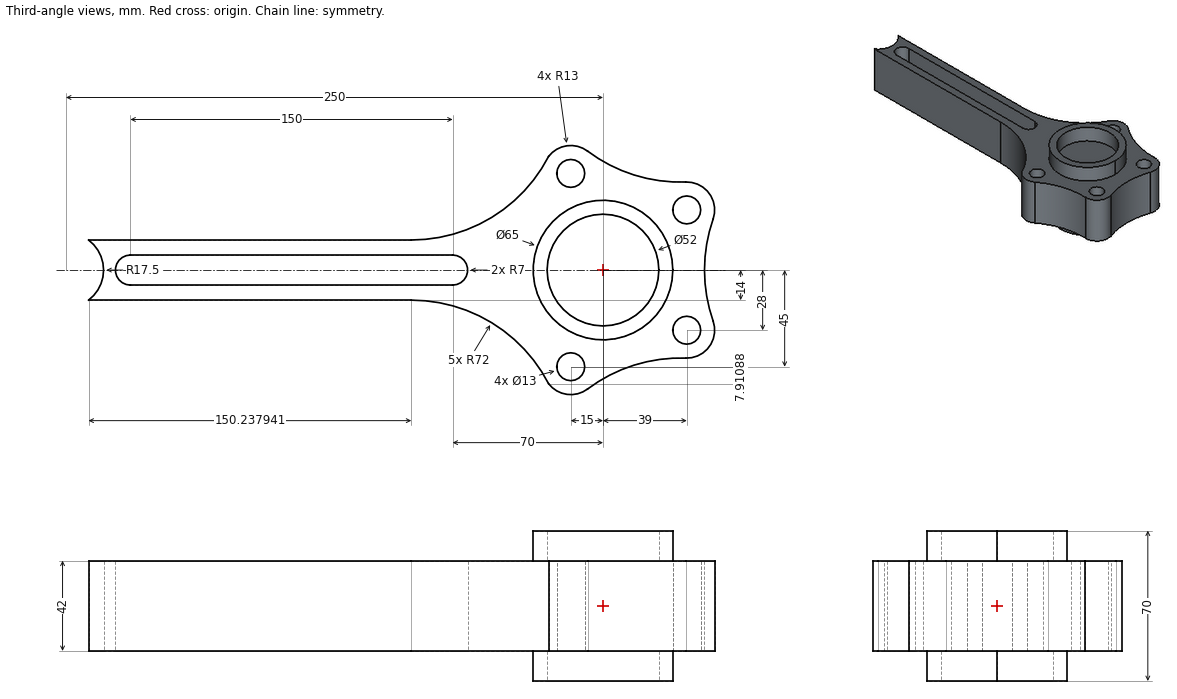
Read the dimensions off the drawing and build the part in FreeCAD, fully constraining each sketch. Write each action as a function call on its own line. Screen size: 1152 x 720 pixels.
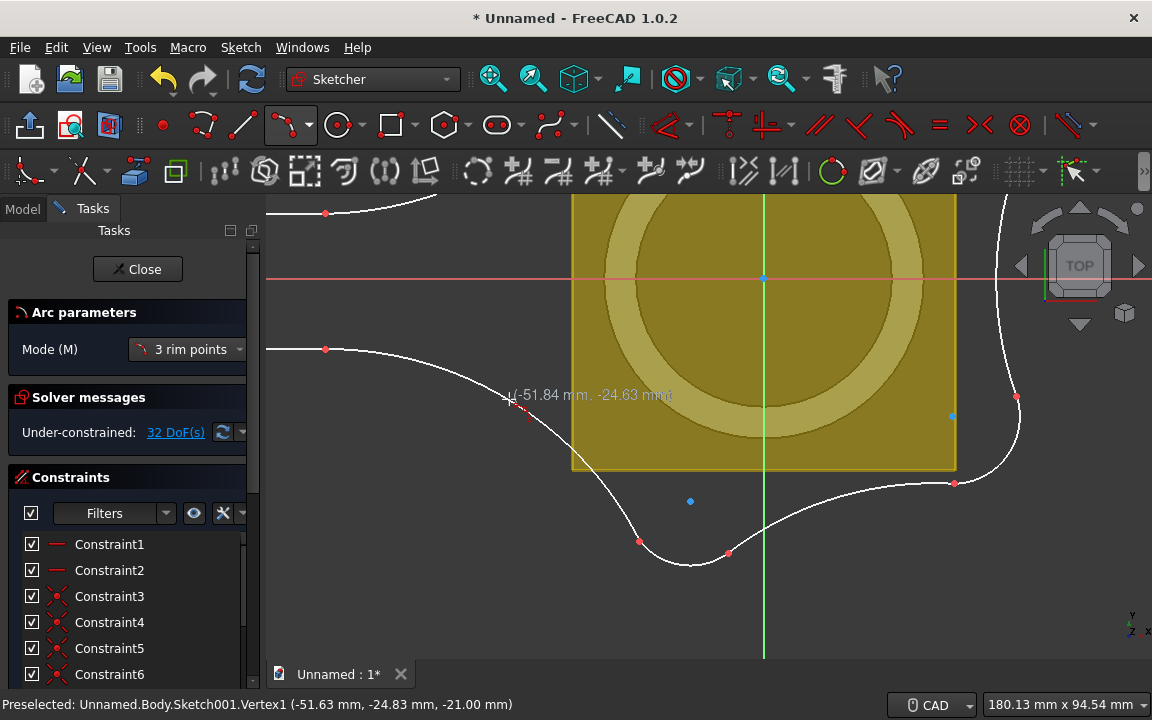
click(498, 126)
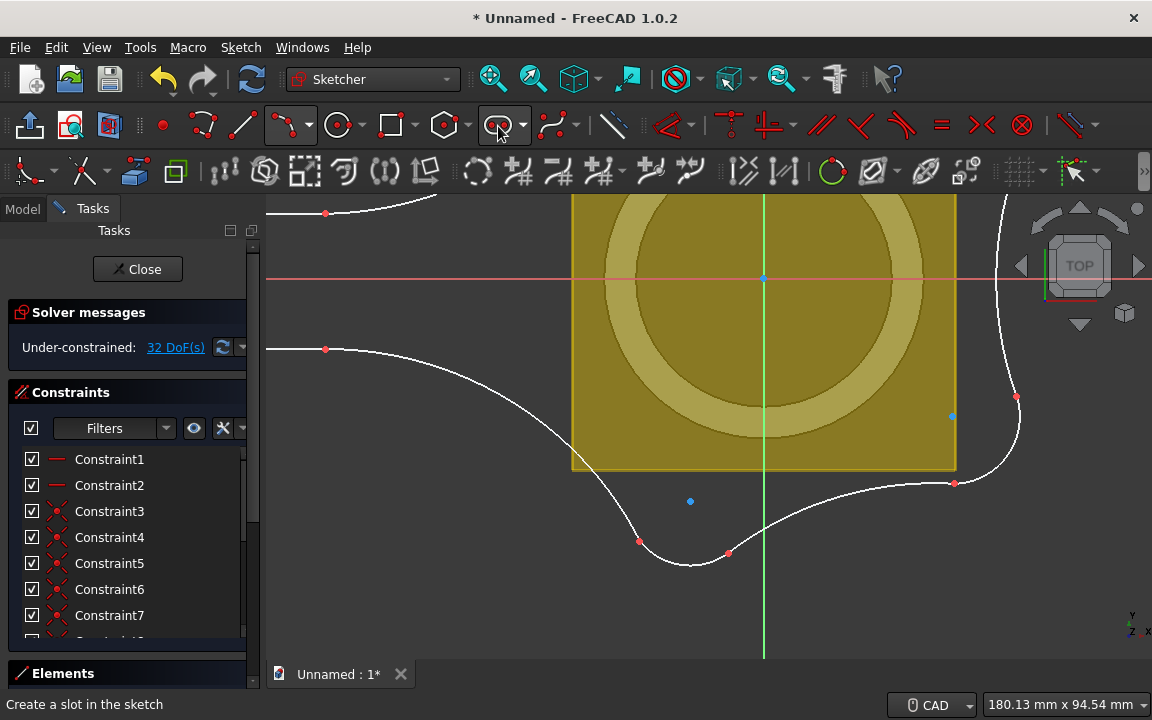
scroll(838, 512, down, 5)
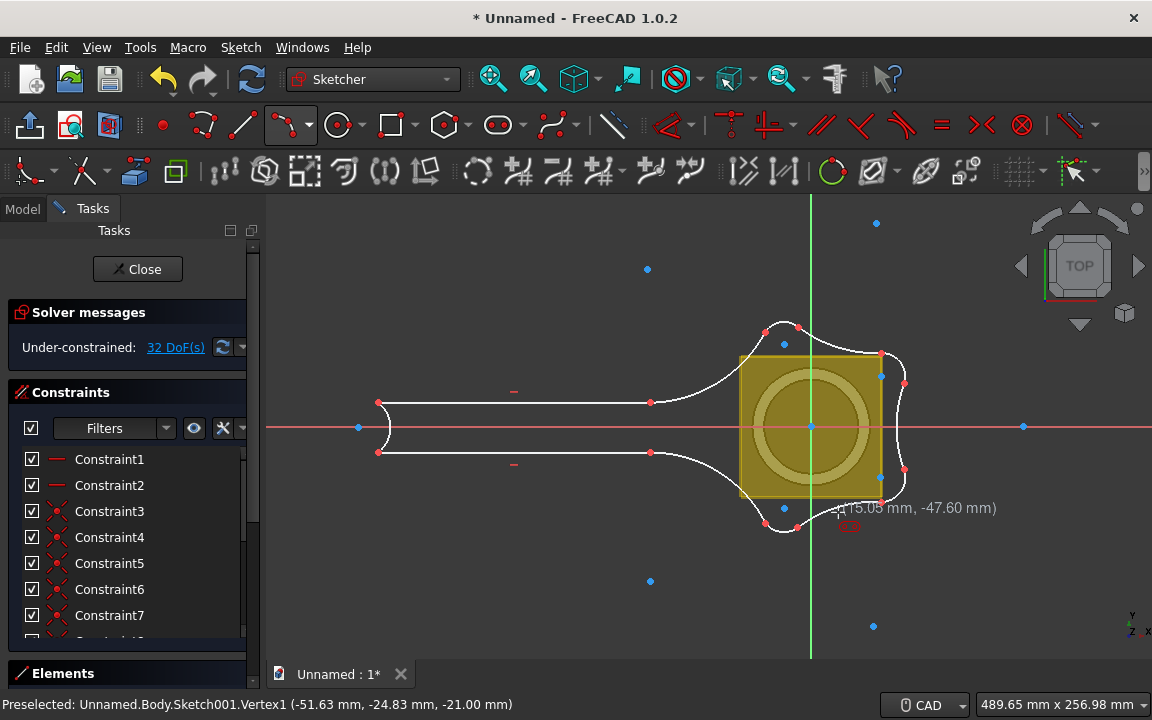
scroll(413, 427, up, 3)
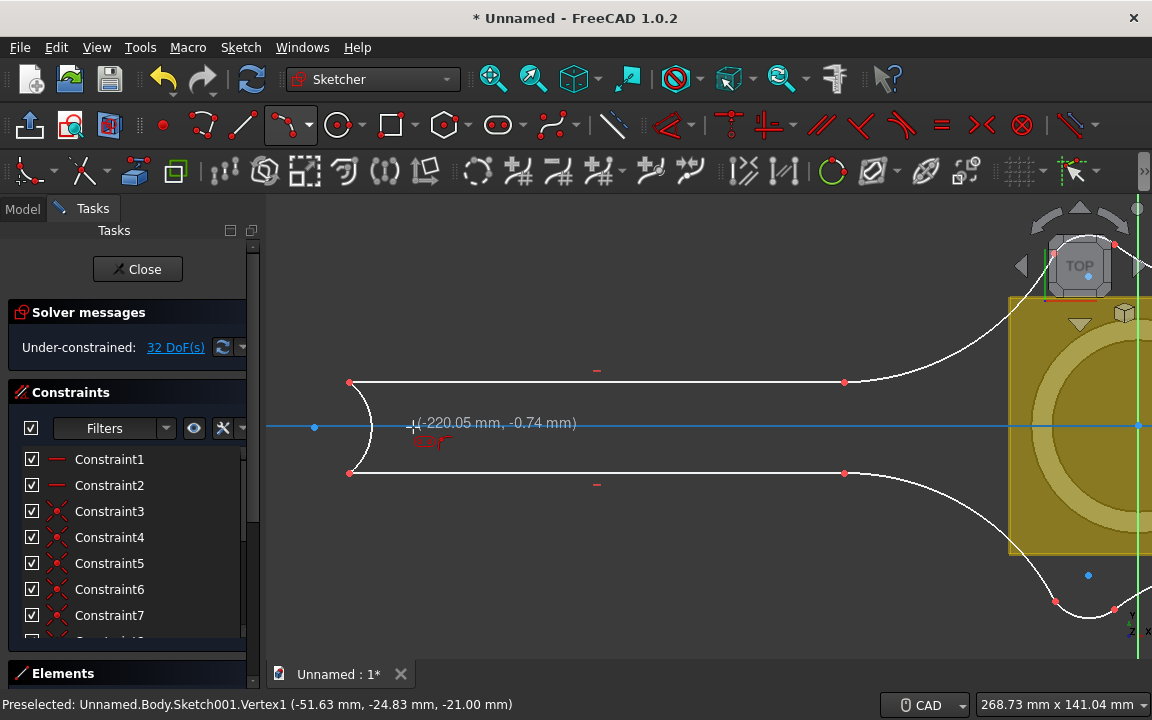
click(413, 426)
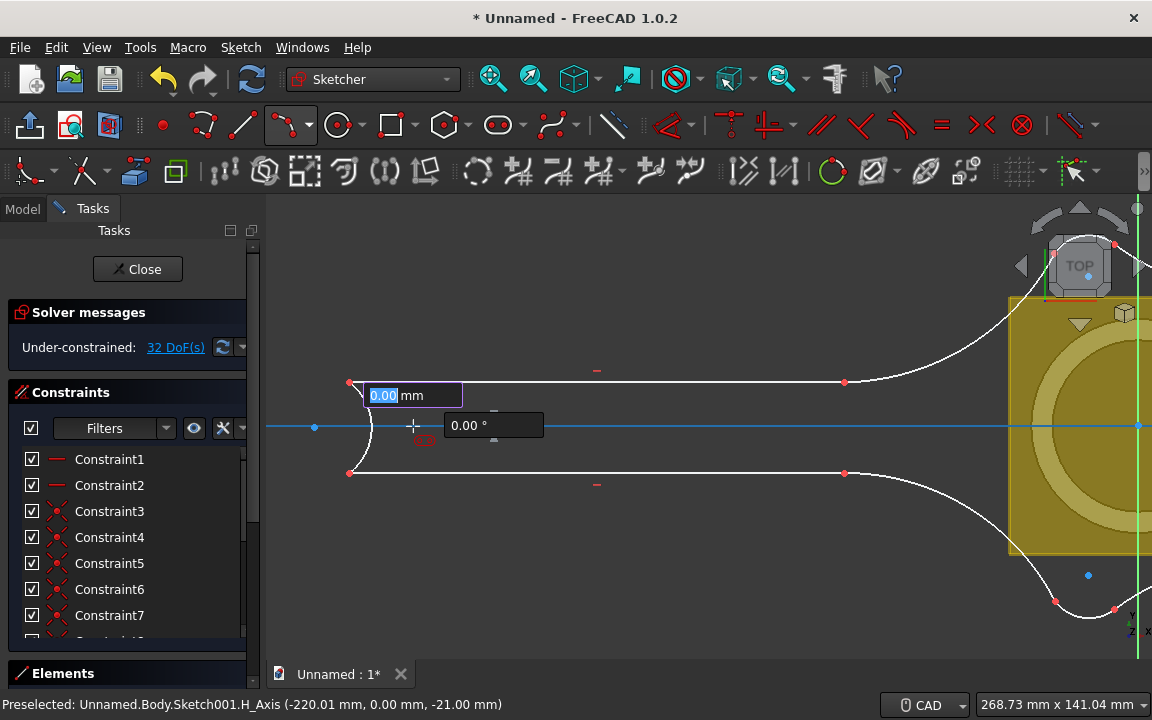
click(908, 417)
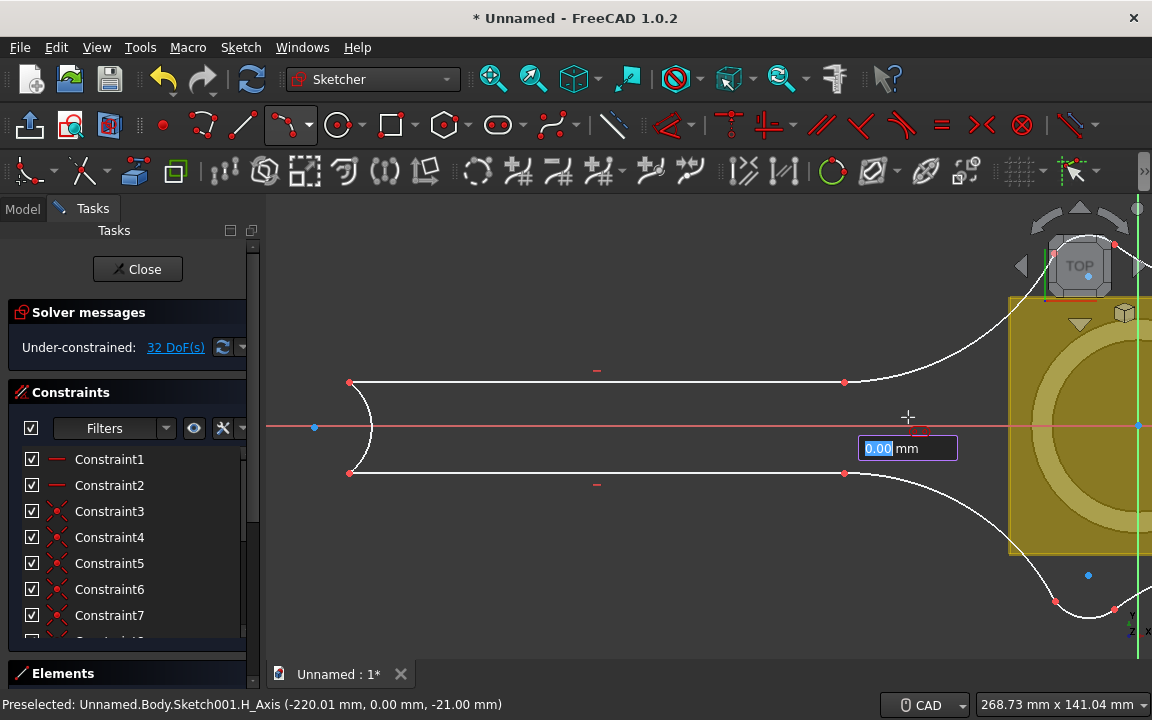
click(660, 449)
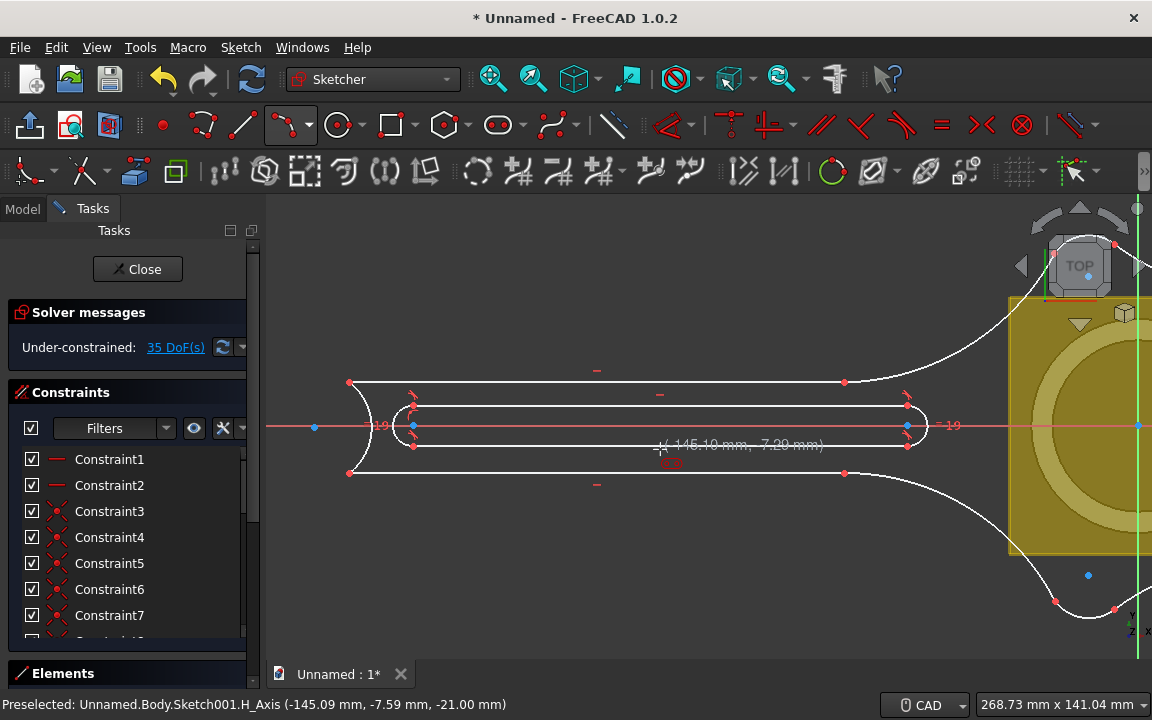
click(338, 126)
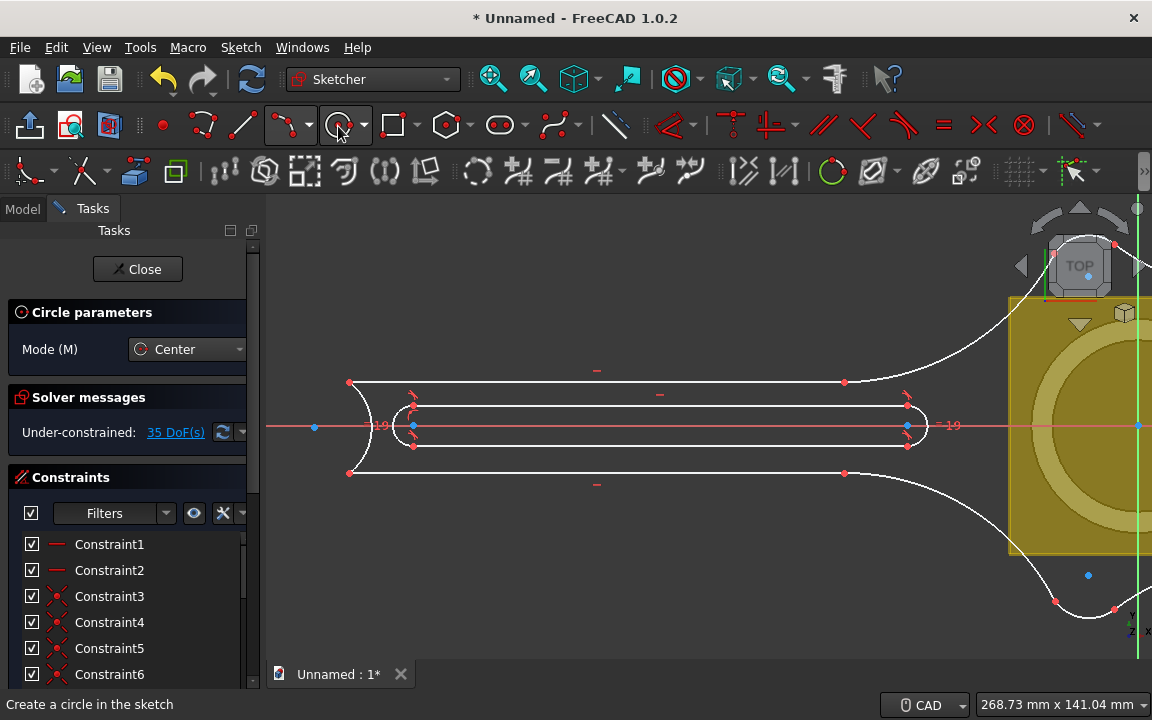
scroll(412, 427, down, 3)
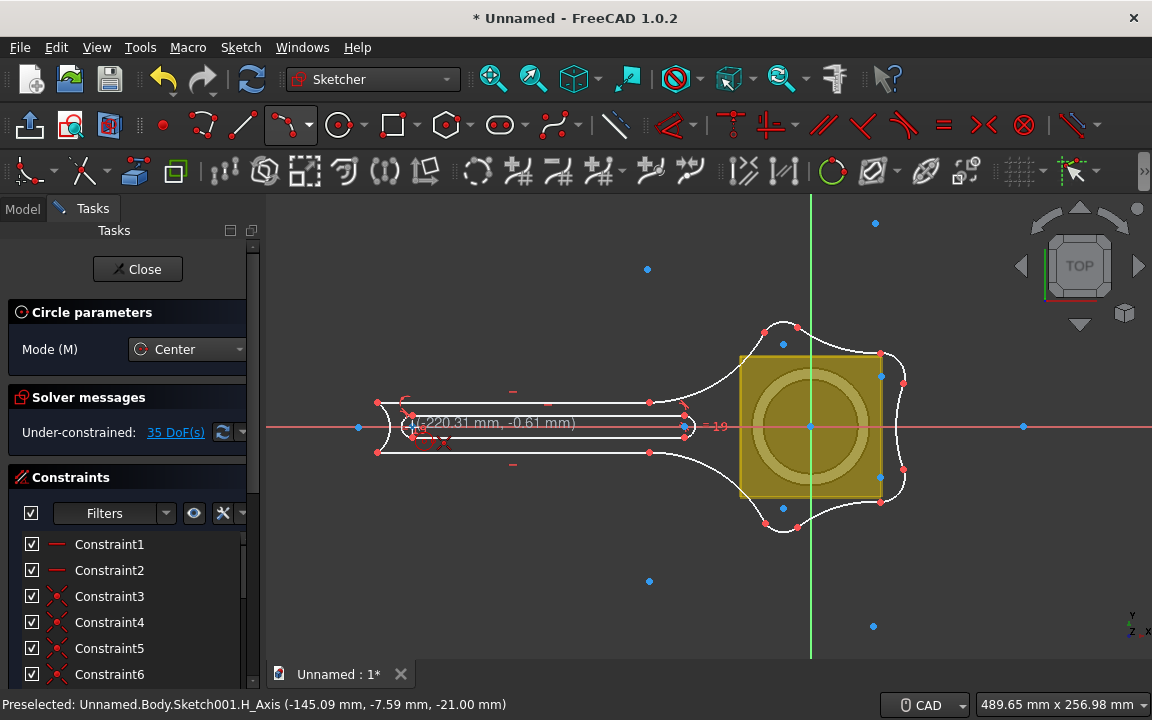
scroll(784, 508, up, 4)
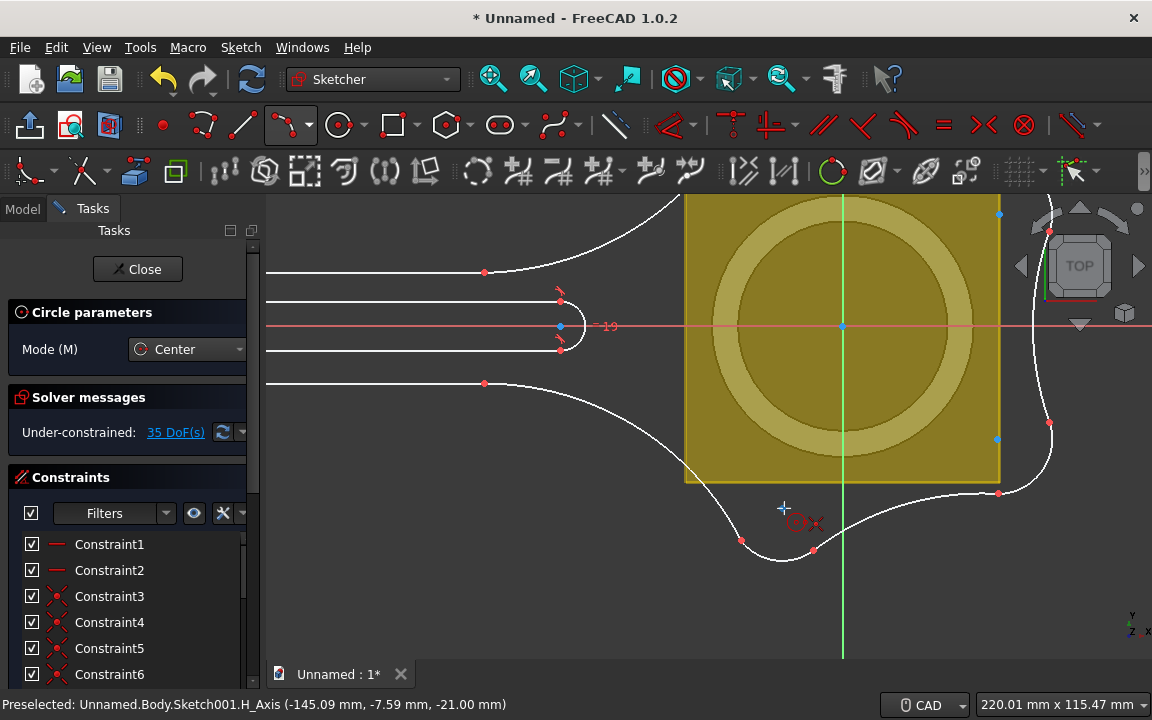
click(782, 507)
move(801, 489)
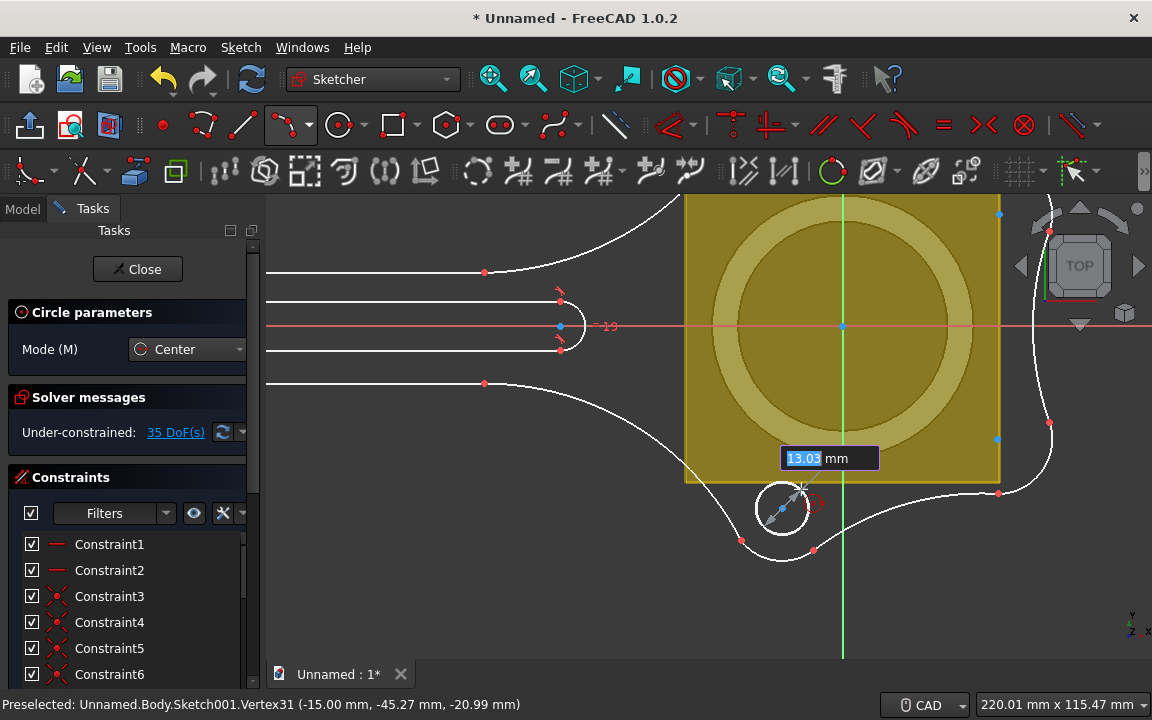
text(13)
key(Return)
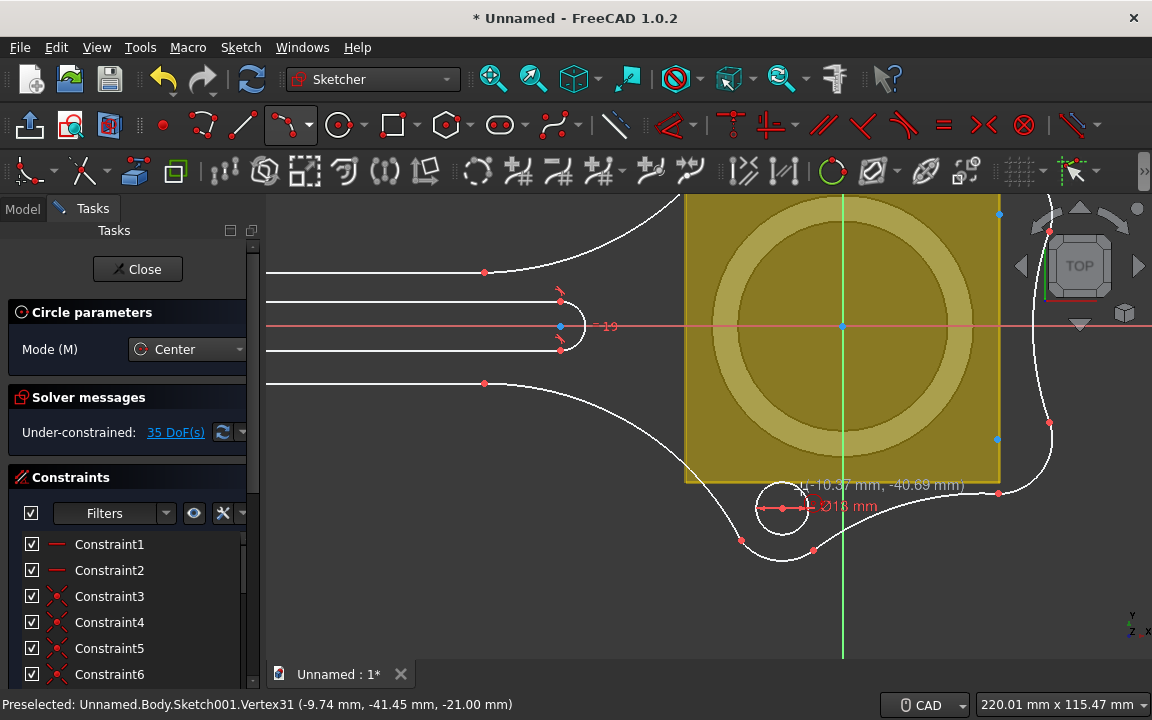
scroll(785, 508, down, 4)